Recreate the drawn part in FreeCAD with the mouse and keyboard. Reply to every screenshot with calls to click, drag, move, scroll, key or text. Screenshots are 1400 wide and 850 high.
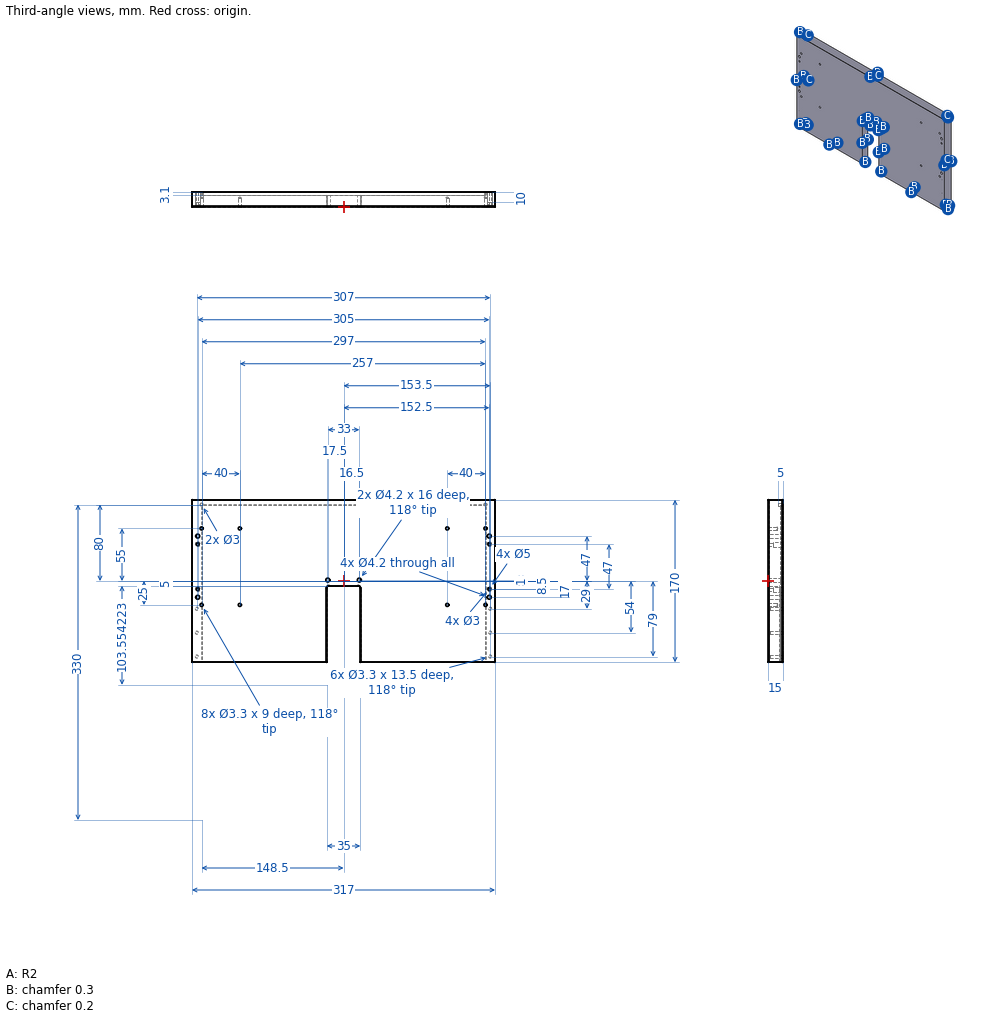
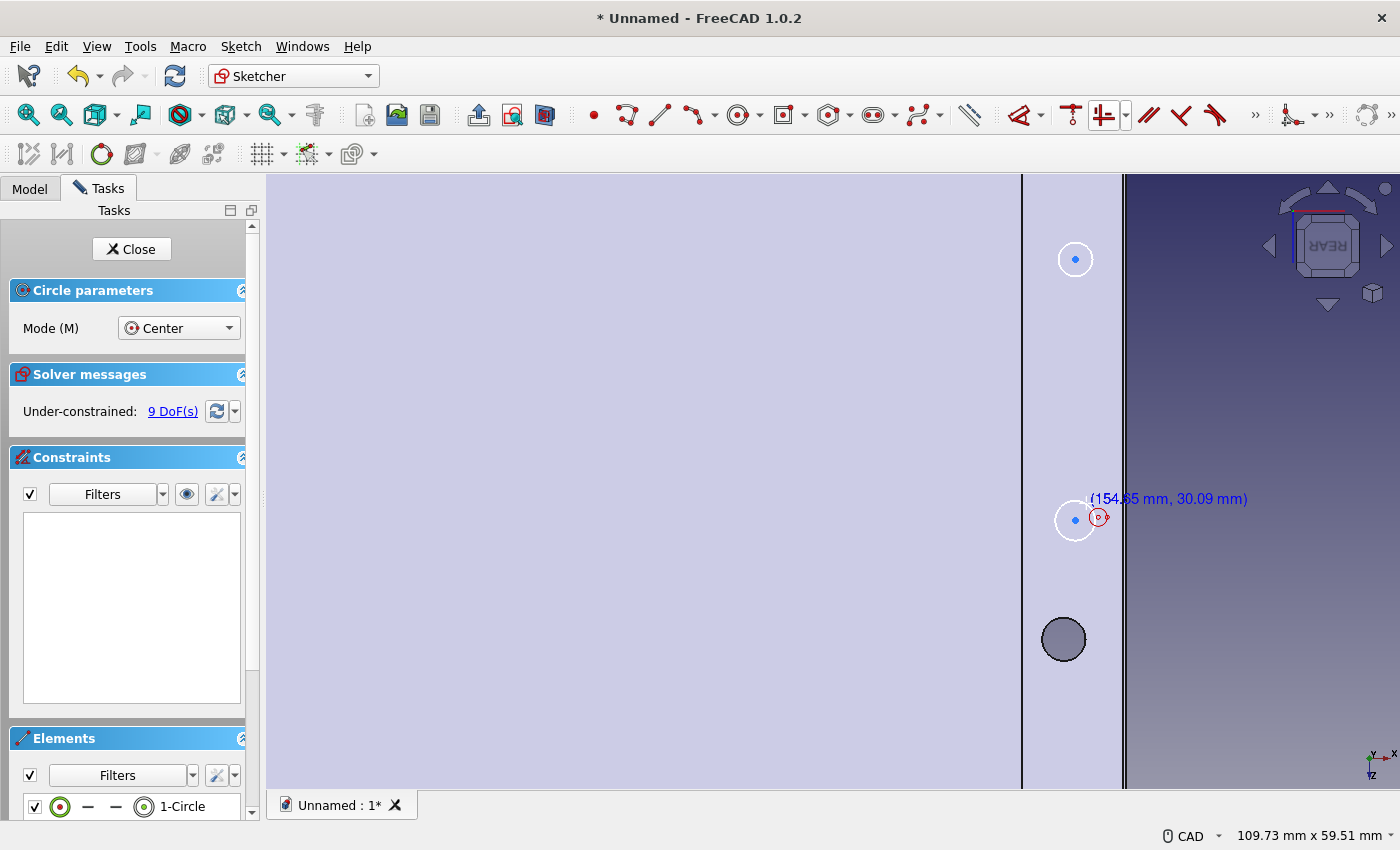
scroll(1087, 503, down, 8)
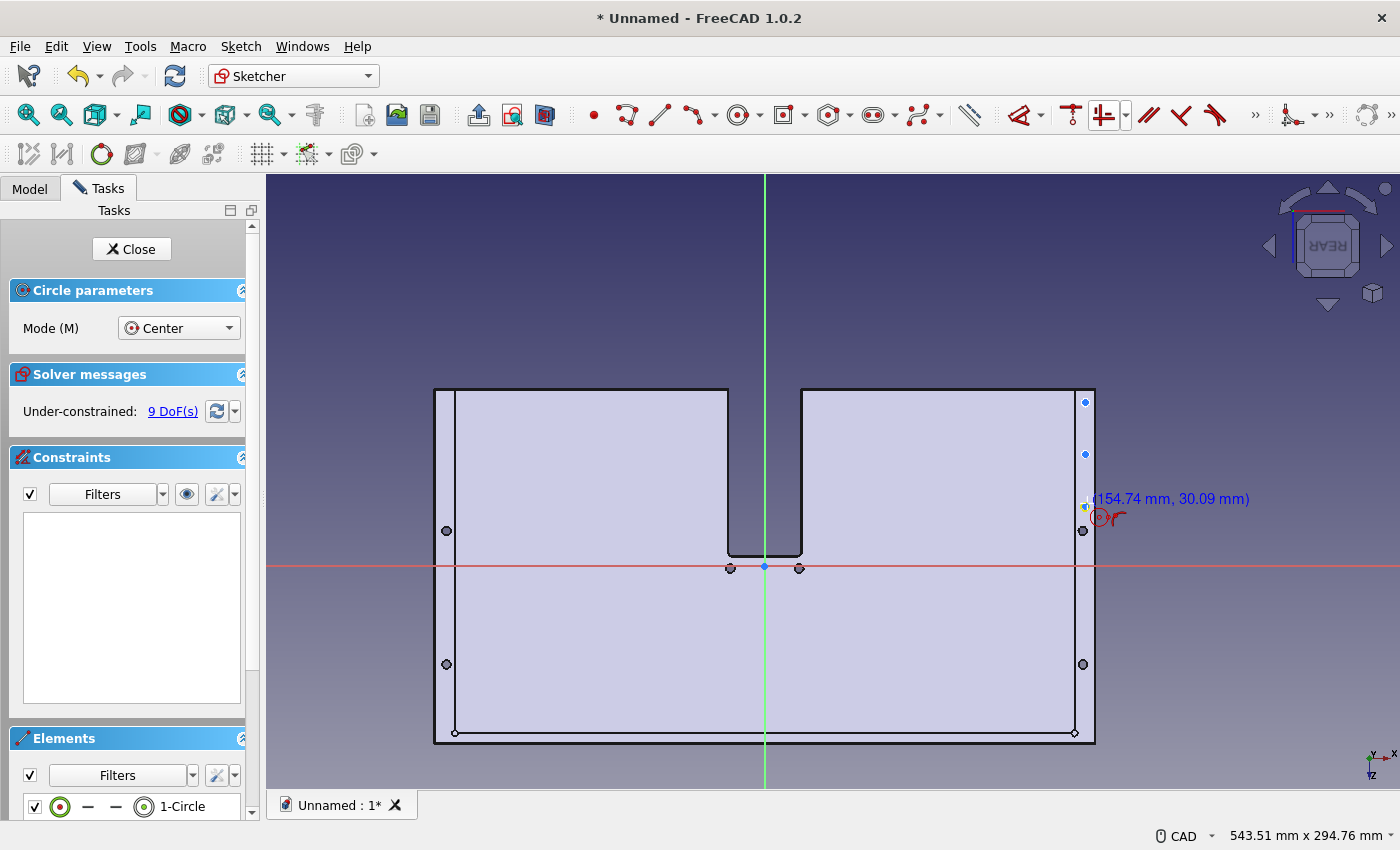
scroll(444, 506, up, 10)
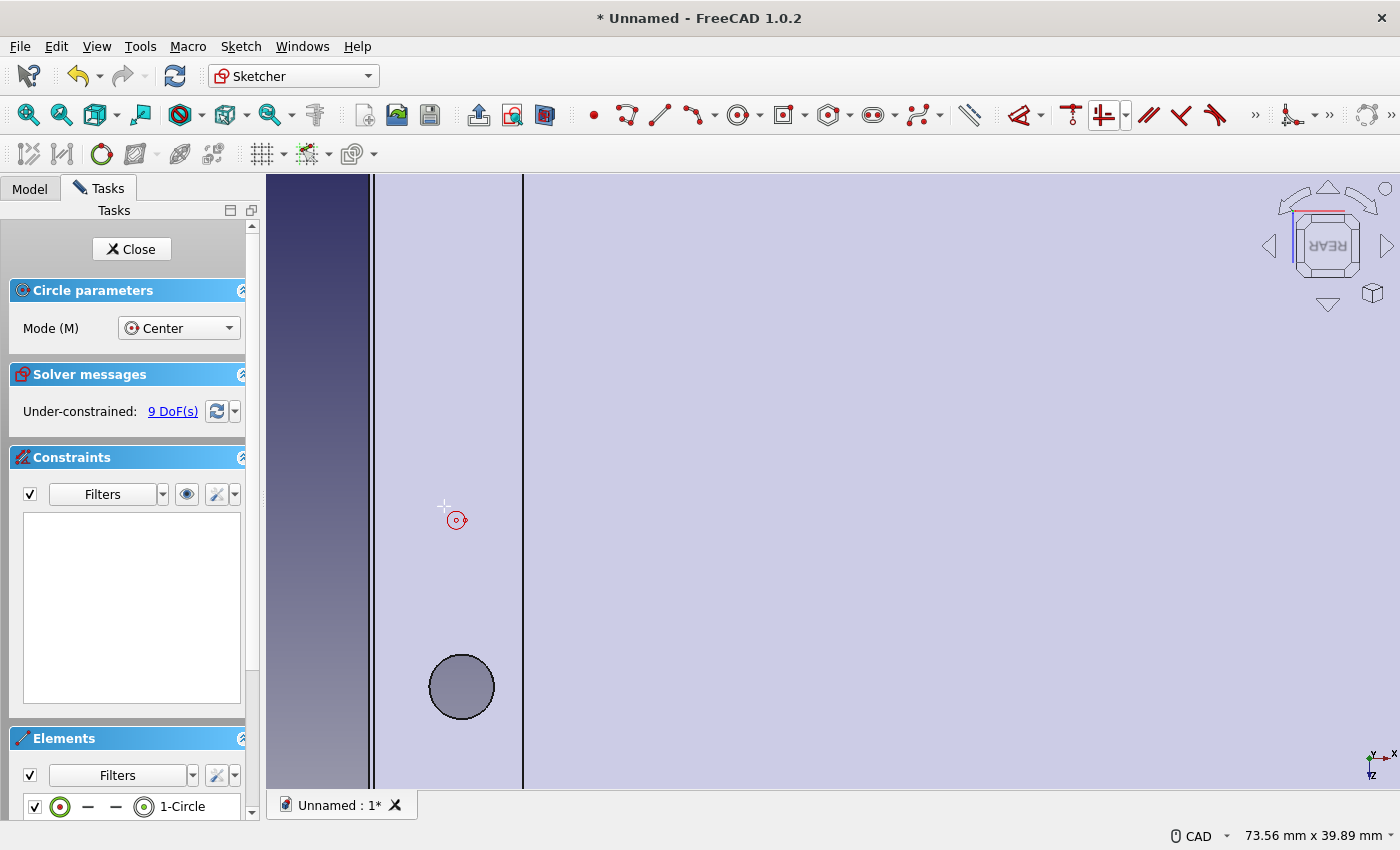
scroll(444, 506, down, 10)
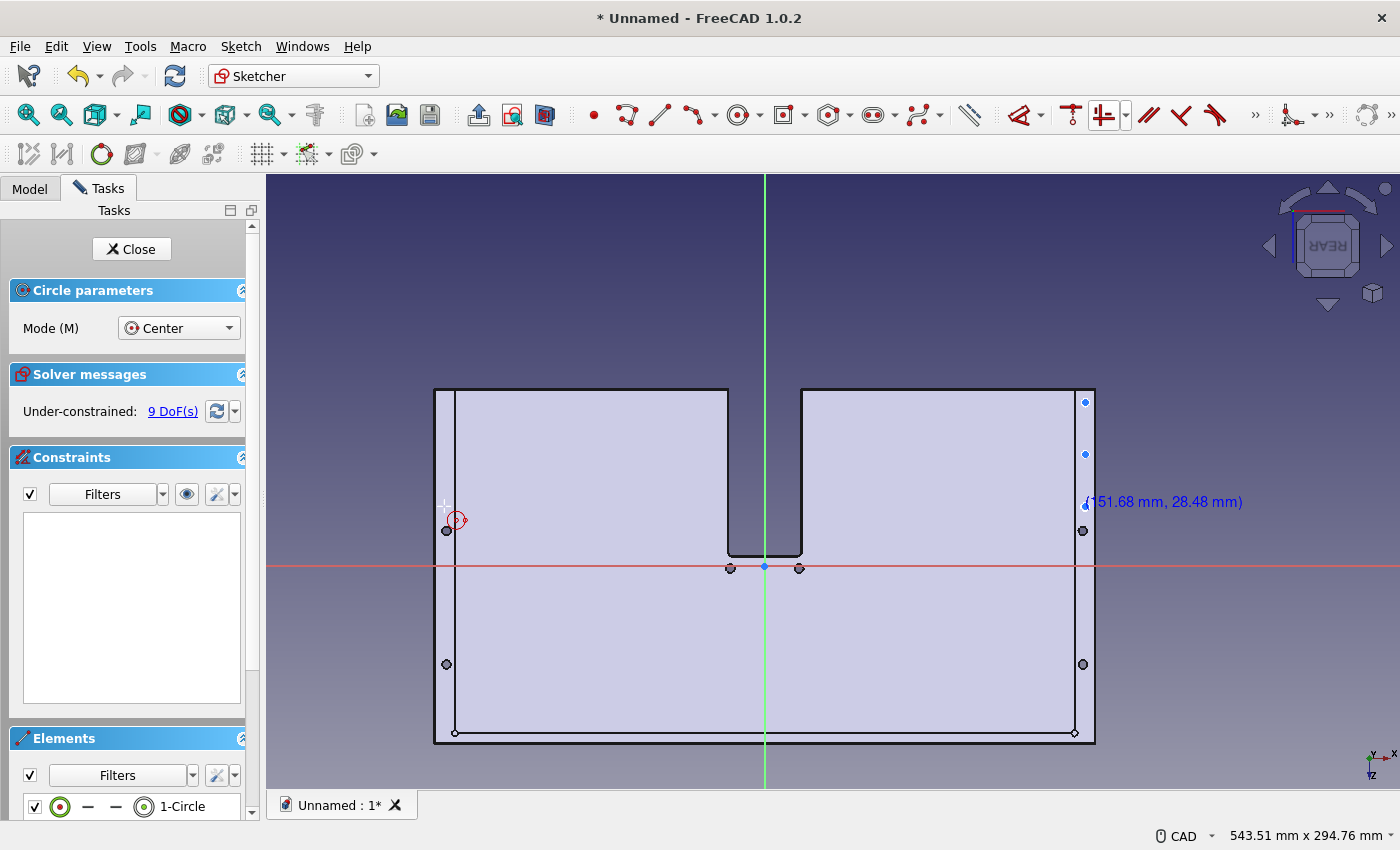
click(444, 506)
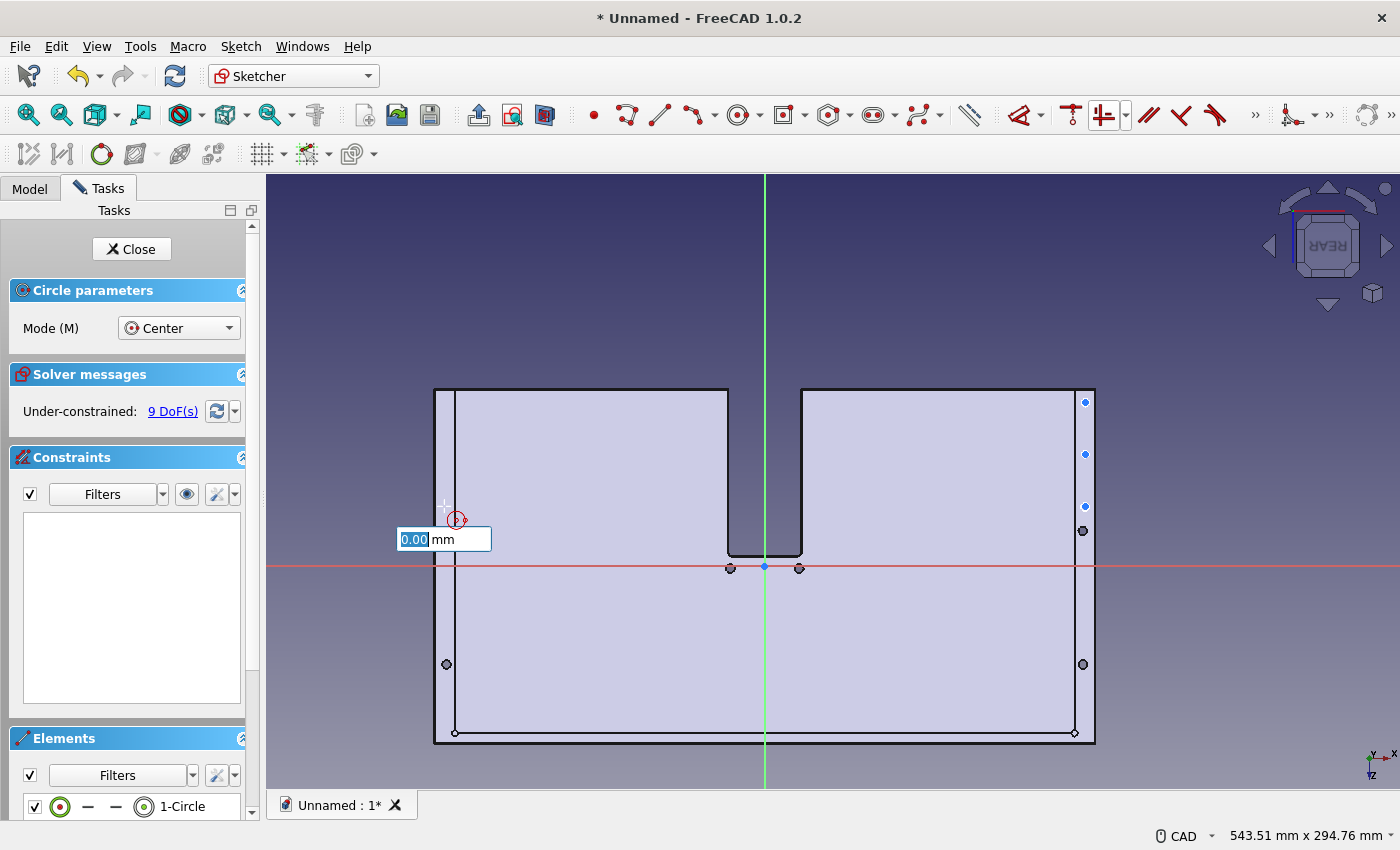
scroll(447, 503, up, 8)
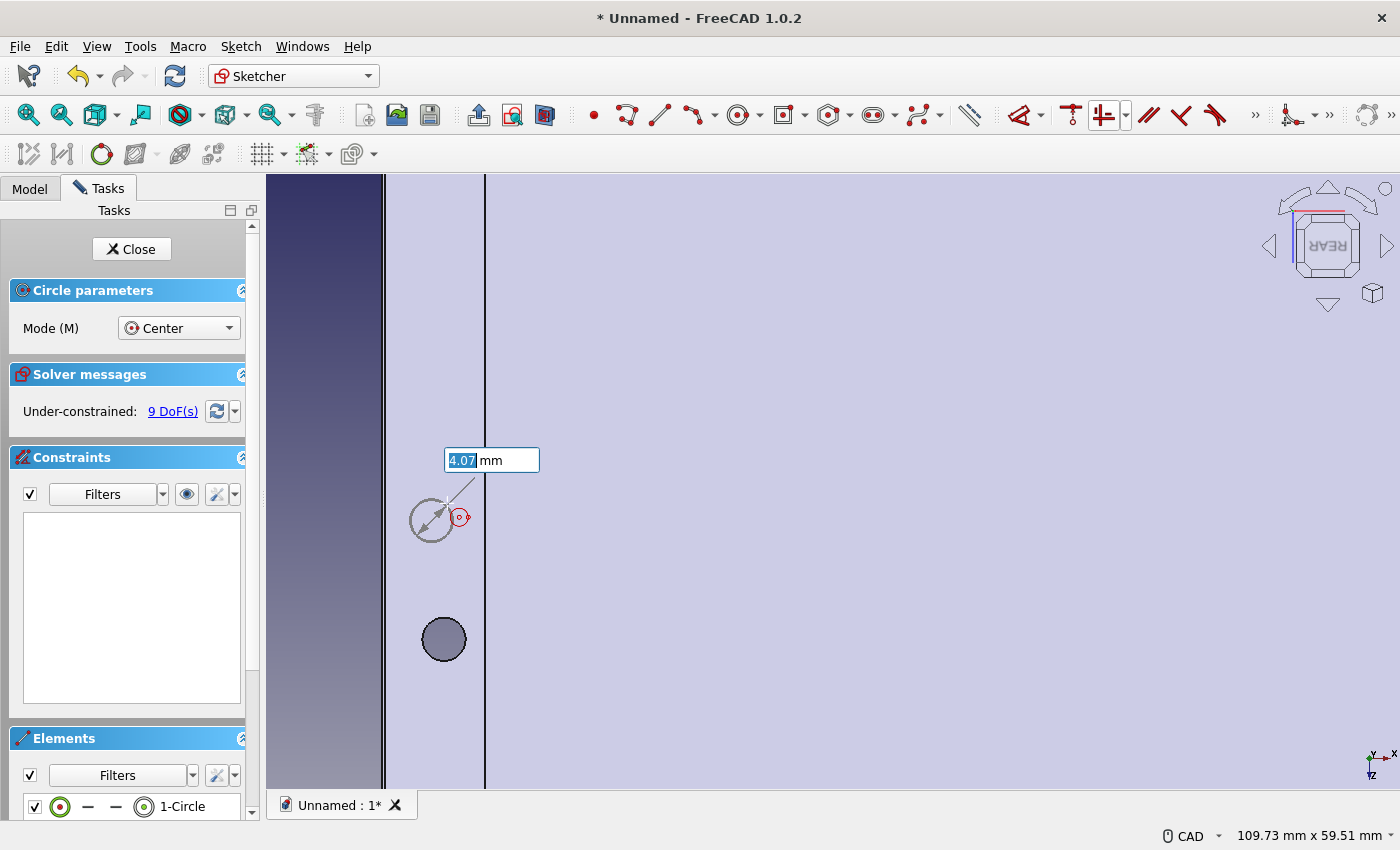
click(446, 503)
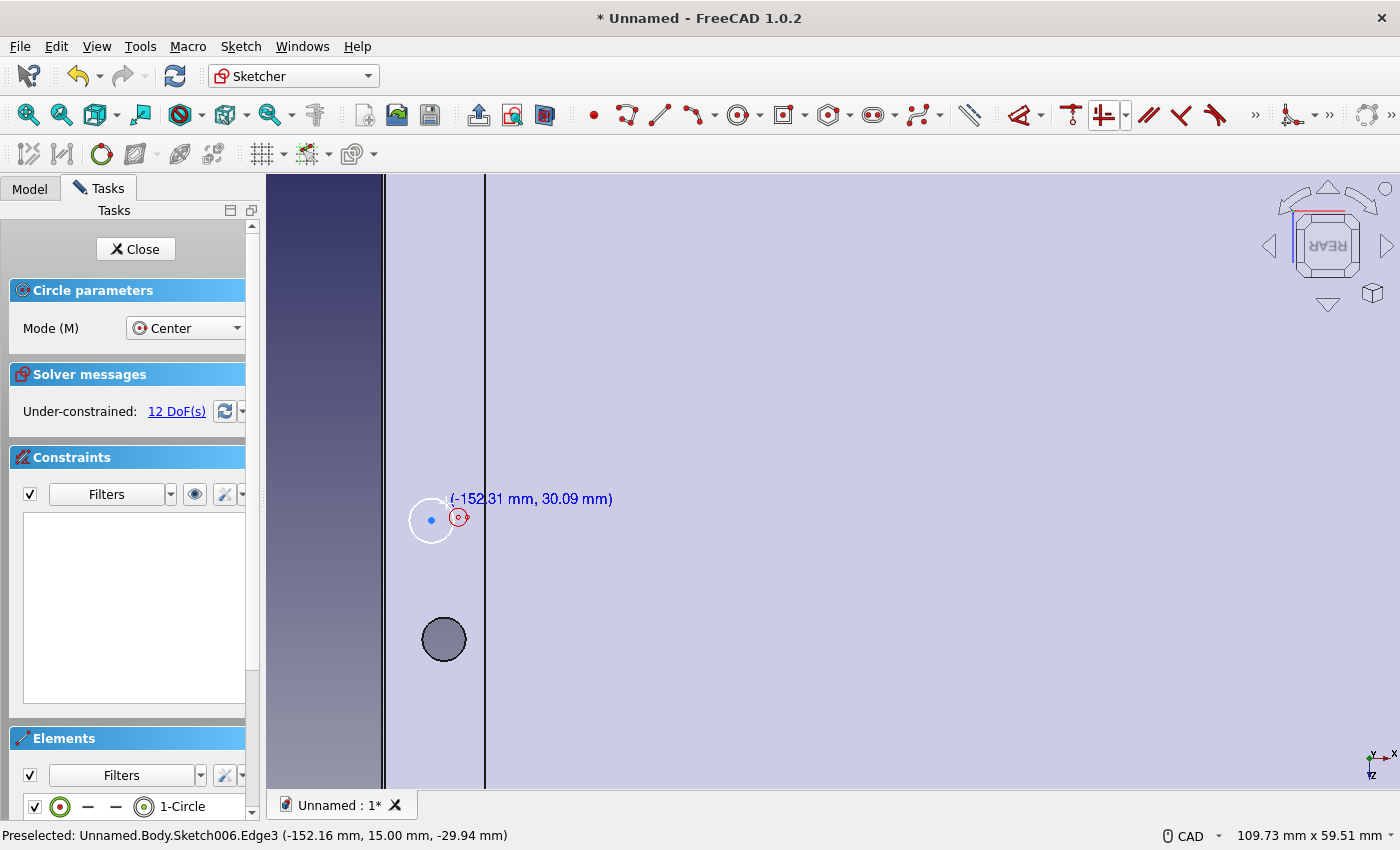
scroll(434, 257, up, 2)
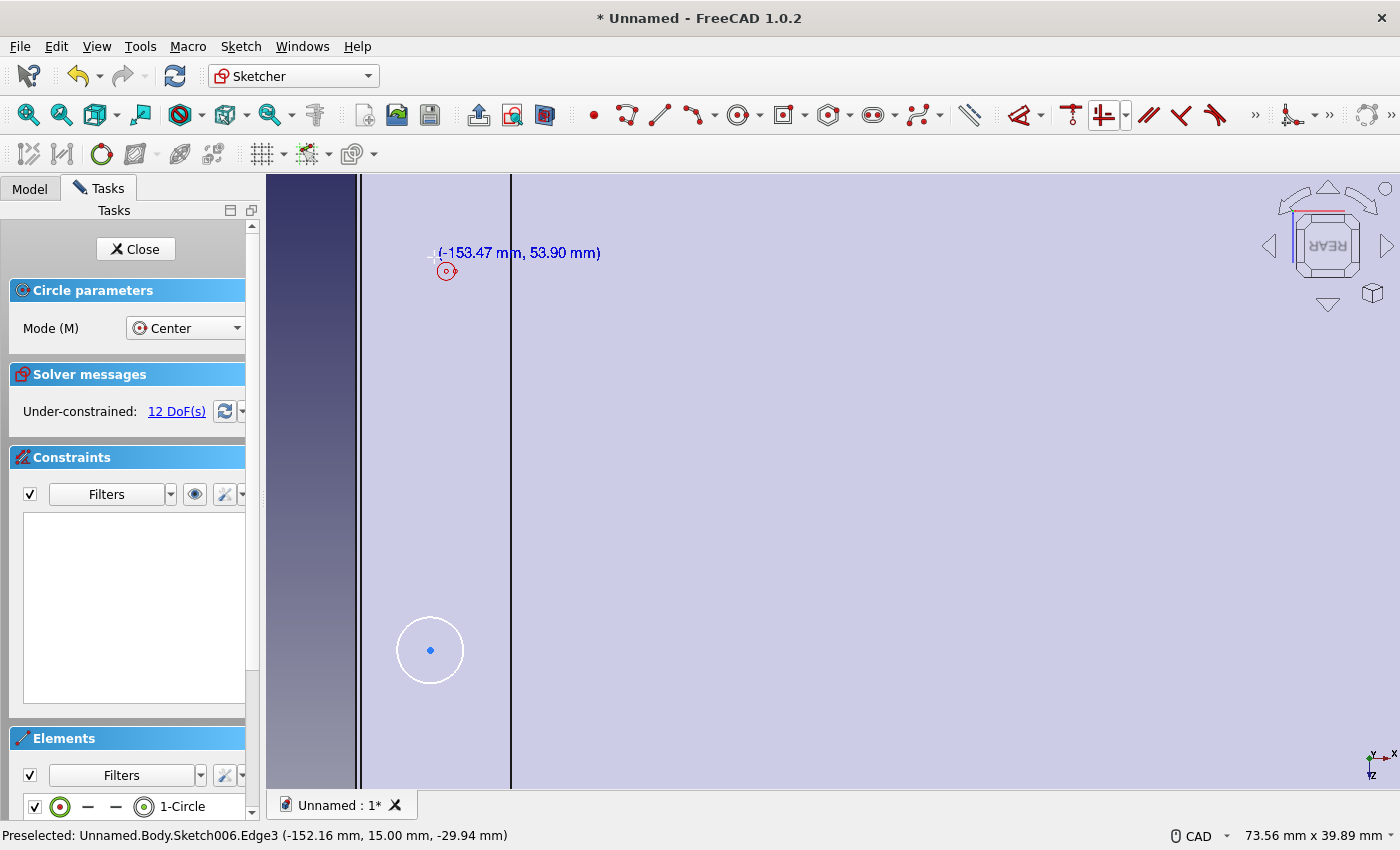
scroll(446, 484, down, 10)